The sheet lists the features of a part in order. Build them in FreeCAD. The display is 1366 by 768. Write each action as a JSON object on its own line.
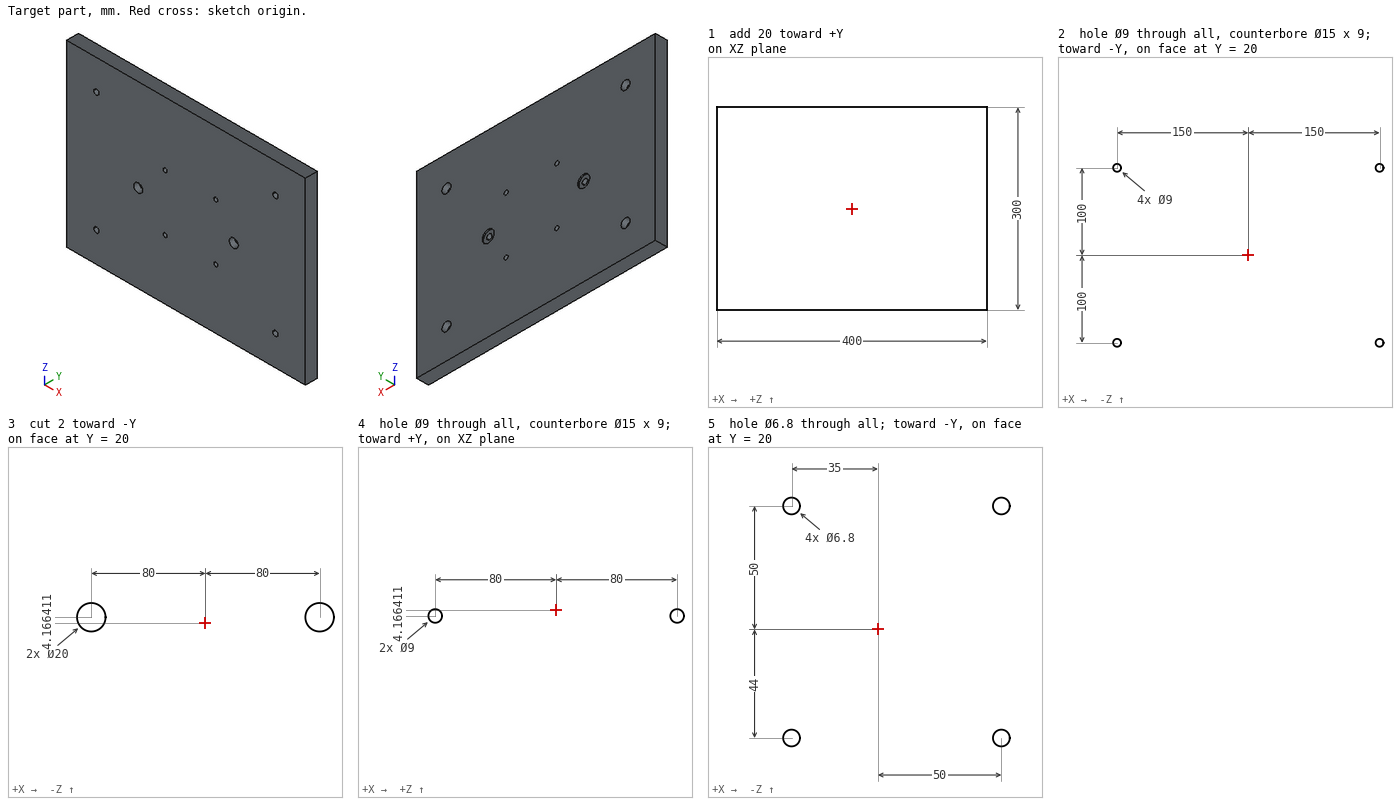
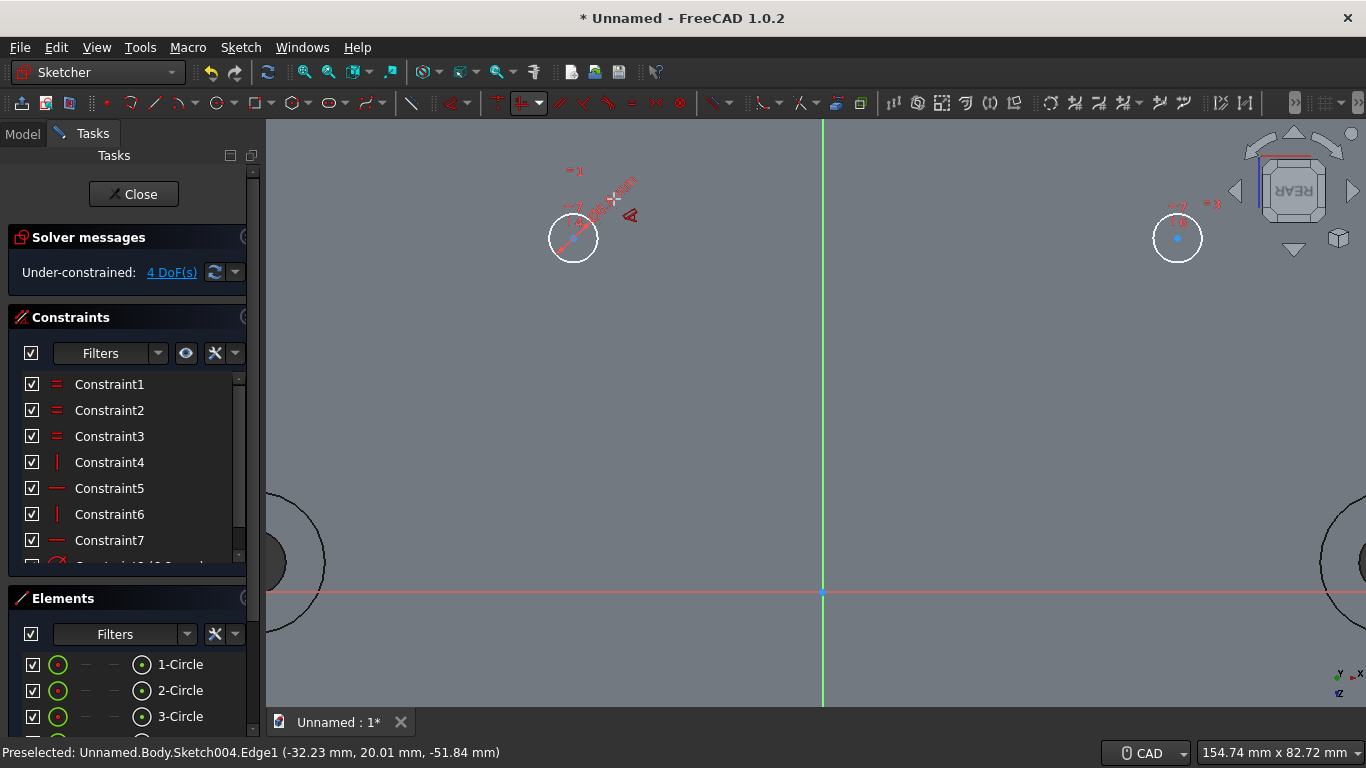
{"action": "left_click", "coordinate": [573, 238]}
{"action": "left_click", "coordinate": [698, 204]}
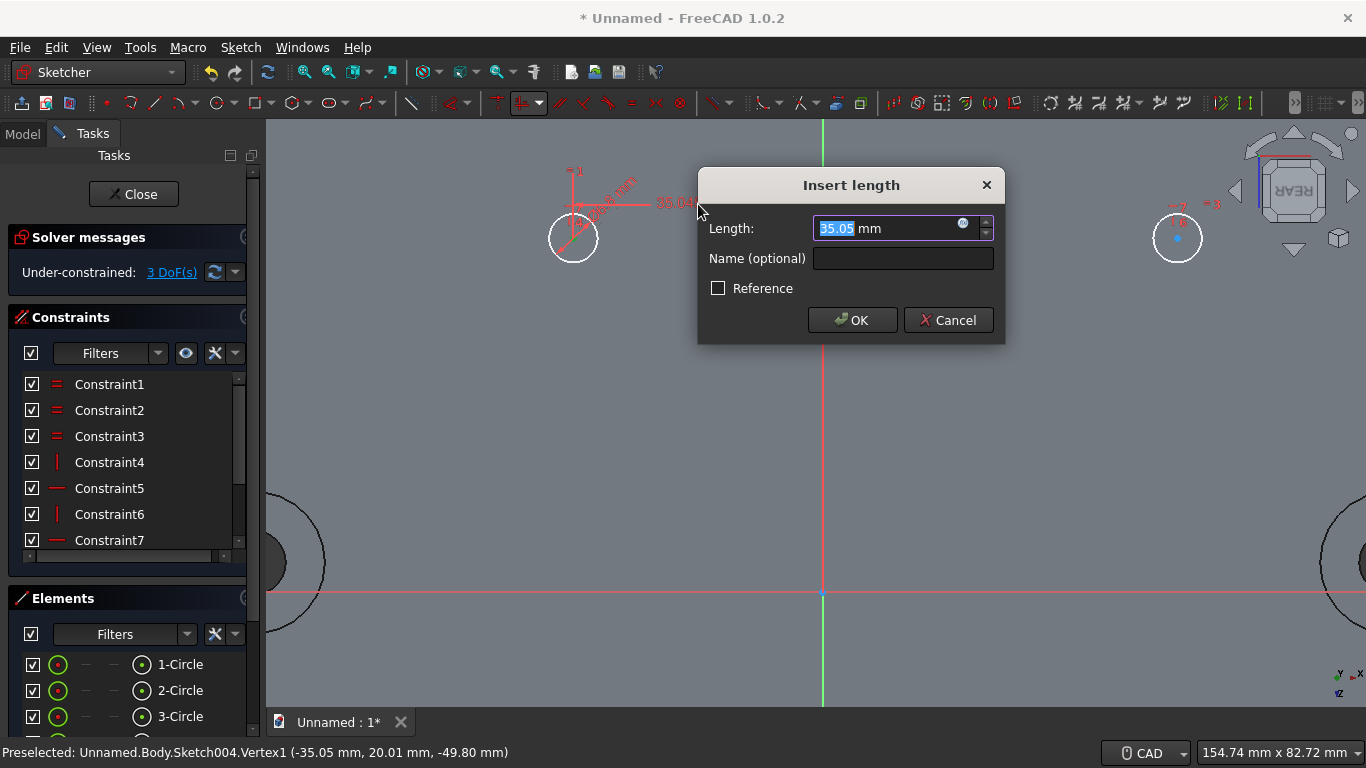
{"action": "type", "text": "35"}
{"action": "key", "text": "Return"}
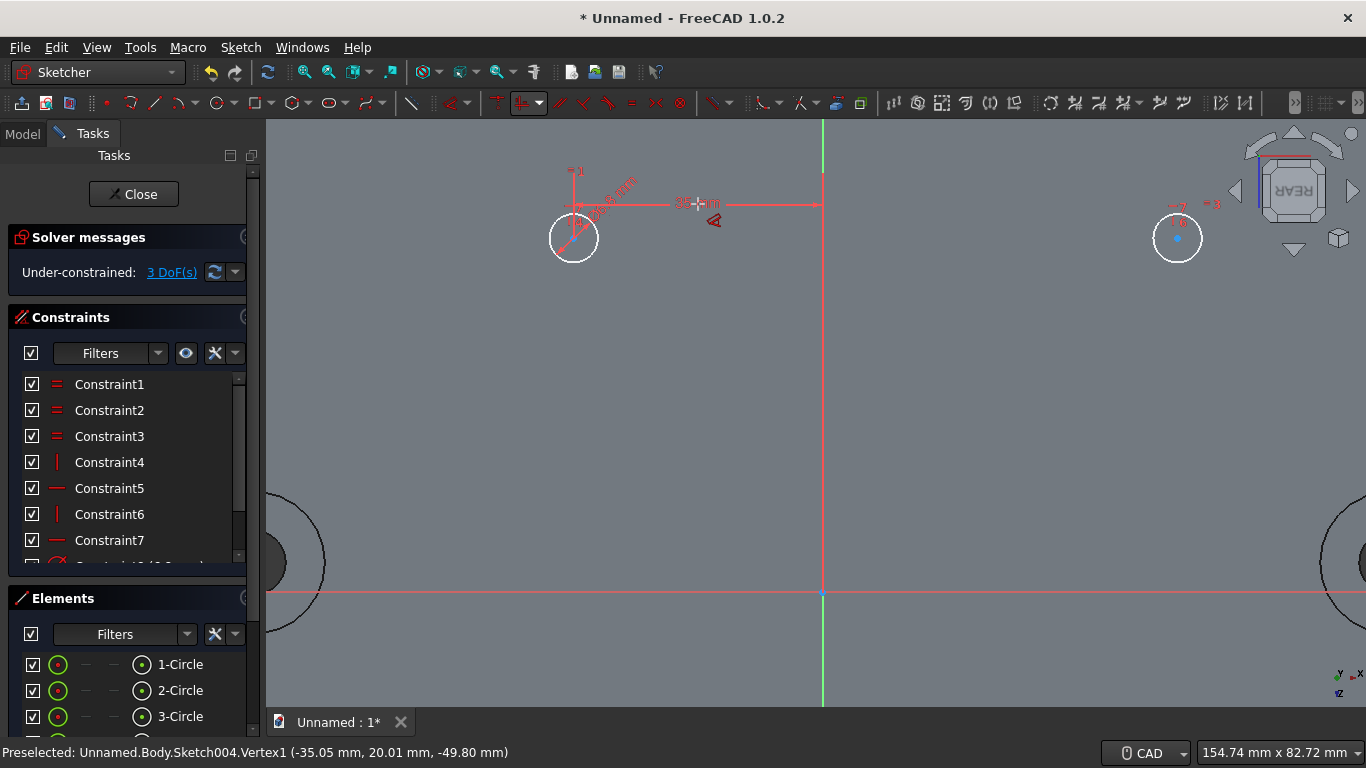
{"action": "left_click", "coordinate": [574, 238]}
{"action": "left_click", "coordinate": [540, 415]}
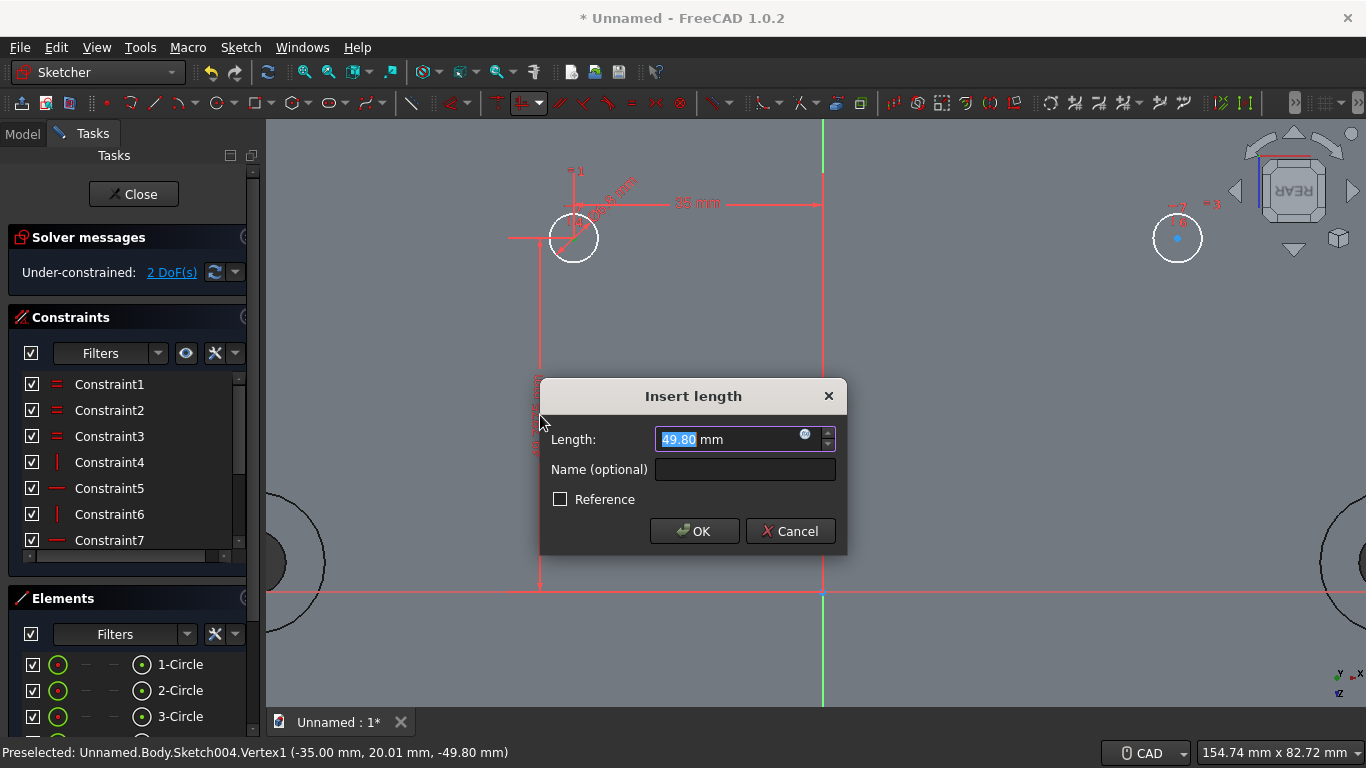
{"action": "type", "text": "50"}
{"action": "key", "text": "Return"}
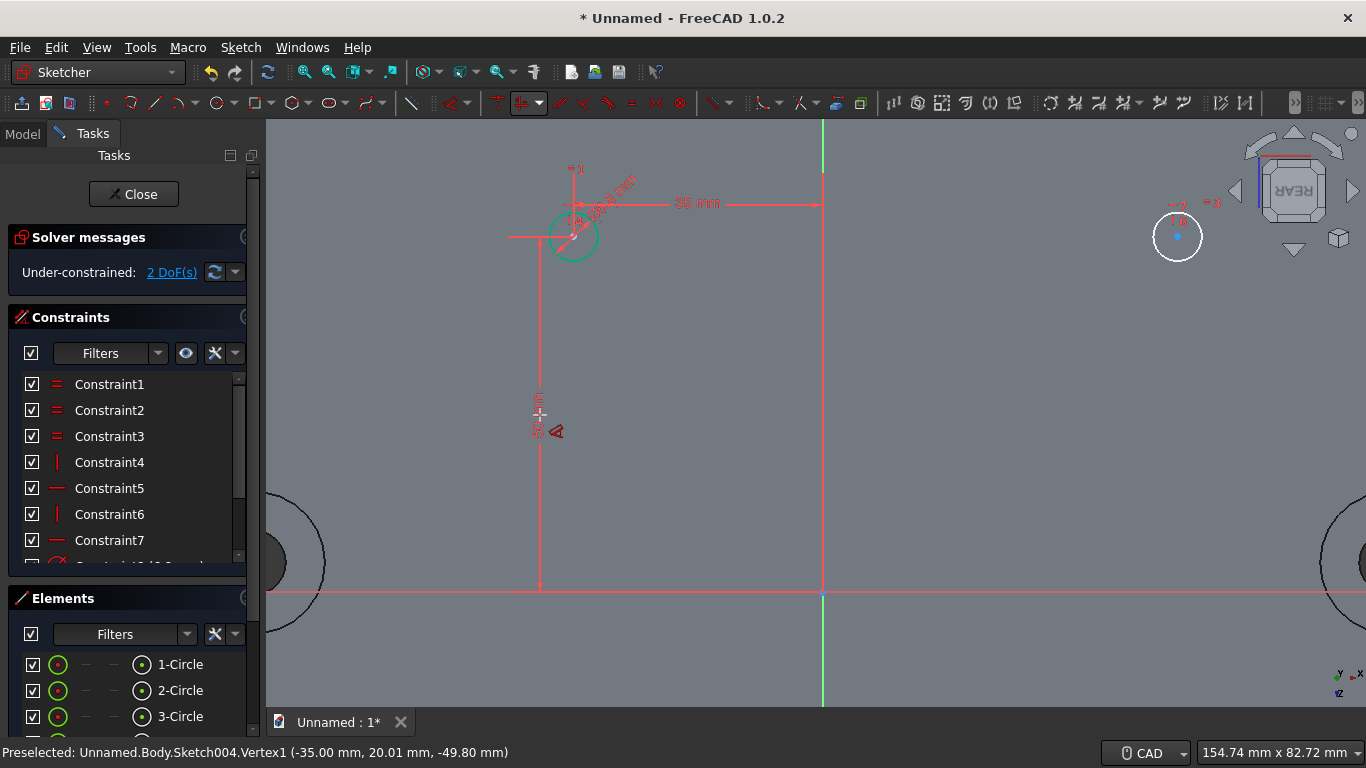
{"action": "scroll", "coordinate": [591, 221], "scroll_direction": "down", "scroll_amount": 3}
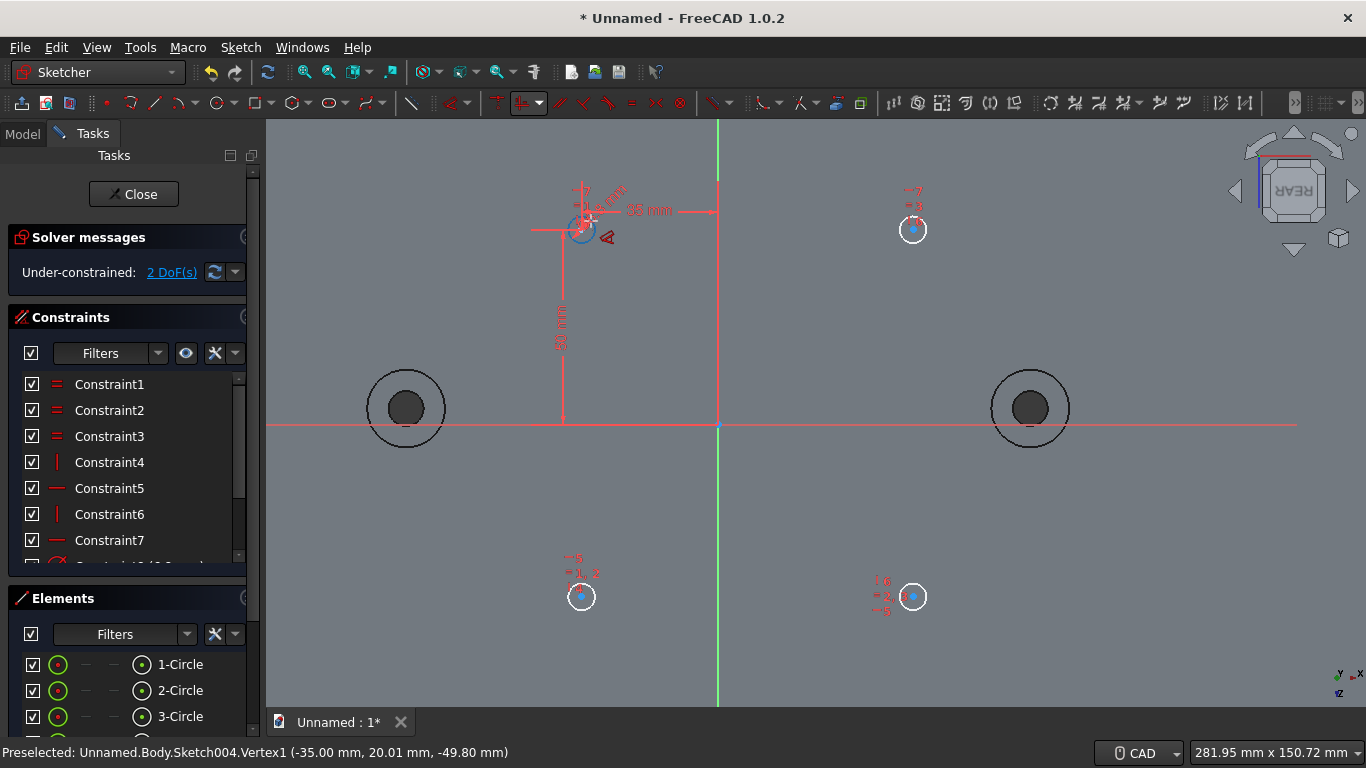
{"action": "left_click", "coordinate": [582, 597]}
{"action": "left_click", "coordinate": [548, 511]}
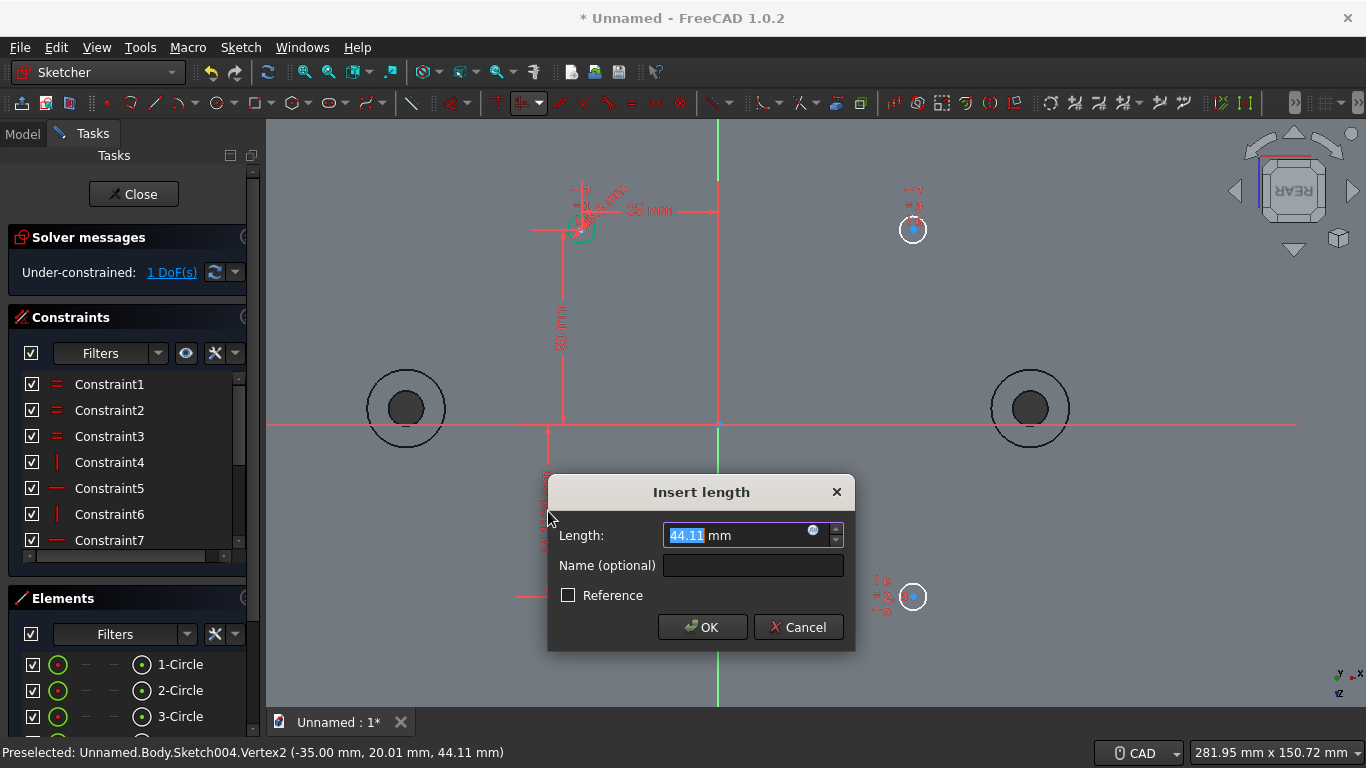
{"action": "type", "text": "44"}
{"action": "key", "text": "Return"}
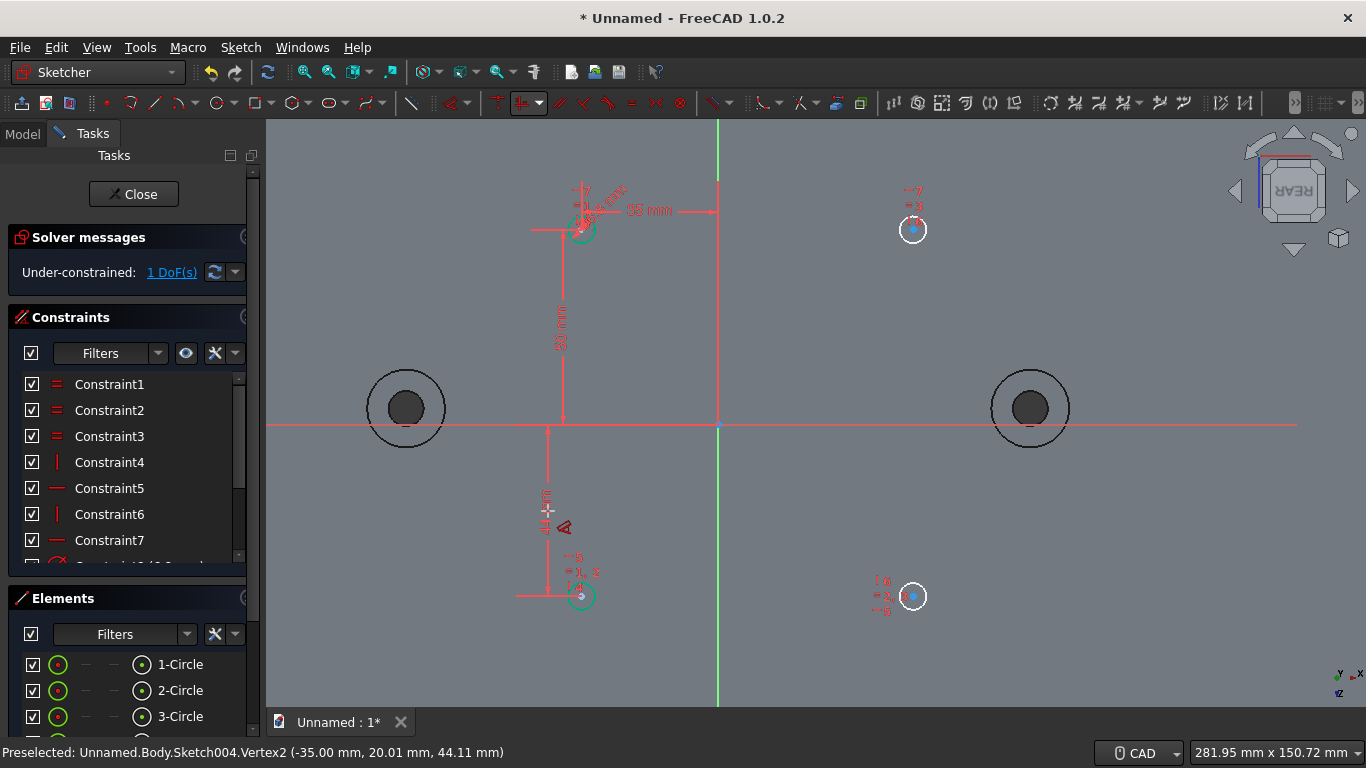
{"action": "left_click", "coordinate": [913, 596]}
{"action": "left_click", "coordinate": [816, 630]}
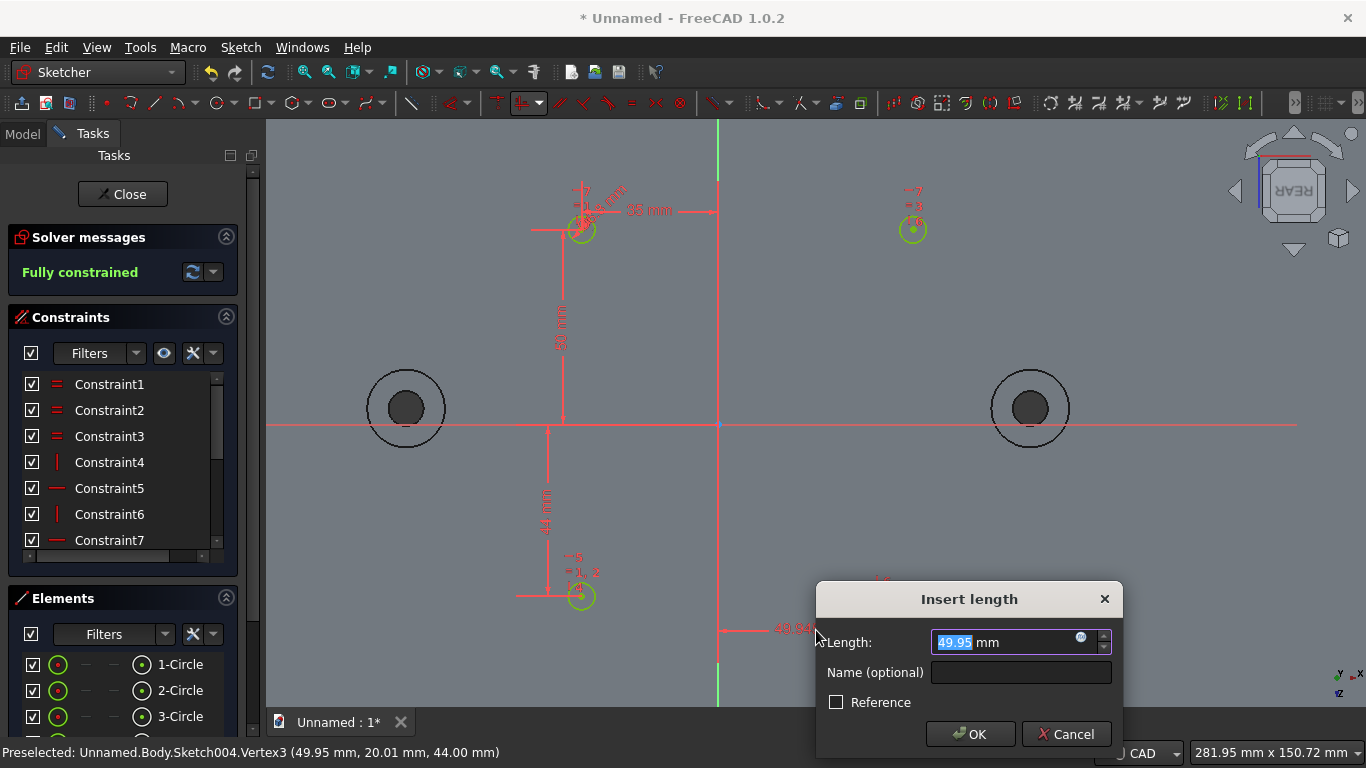
{"action": "type", "text": "50"}
{"action": "key", "text": "Return"}
{"action": "key", "text": "Escape"}